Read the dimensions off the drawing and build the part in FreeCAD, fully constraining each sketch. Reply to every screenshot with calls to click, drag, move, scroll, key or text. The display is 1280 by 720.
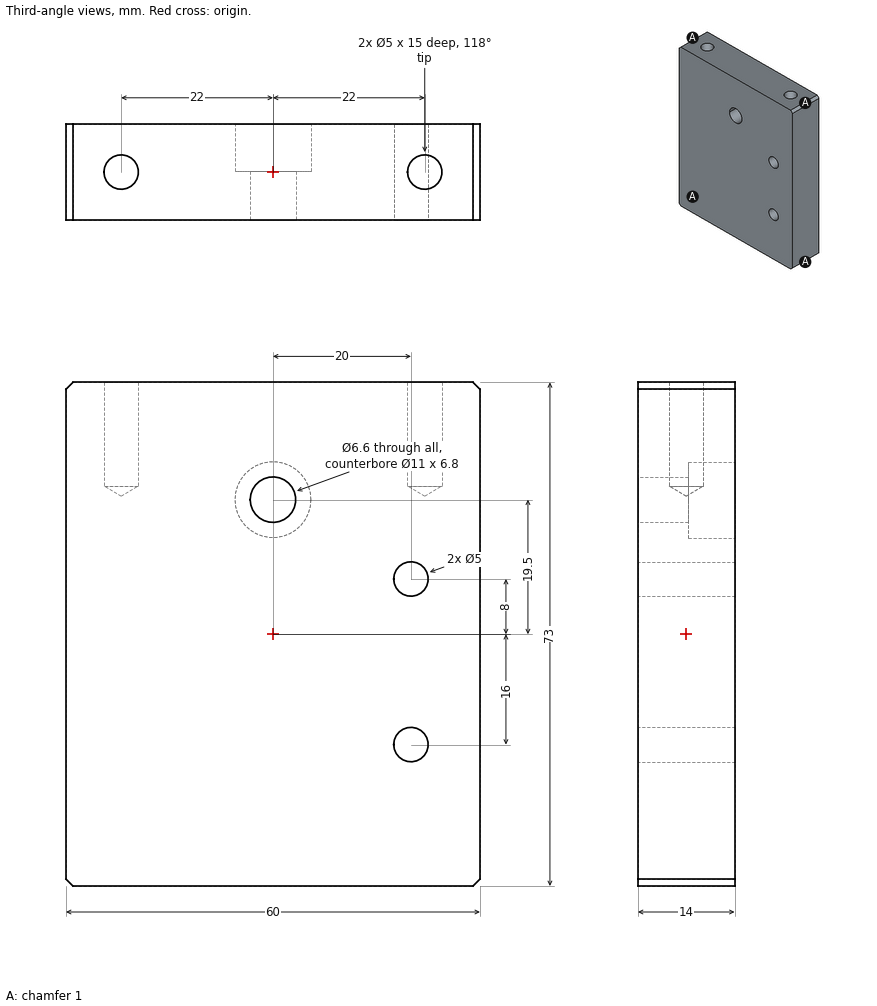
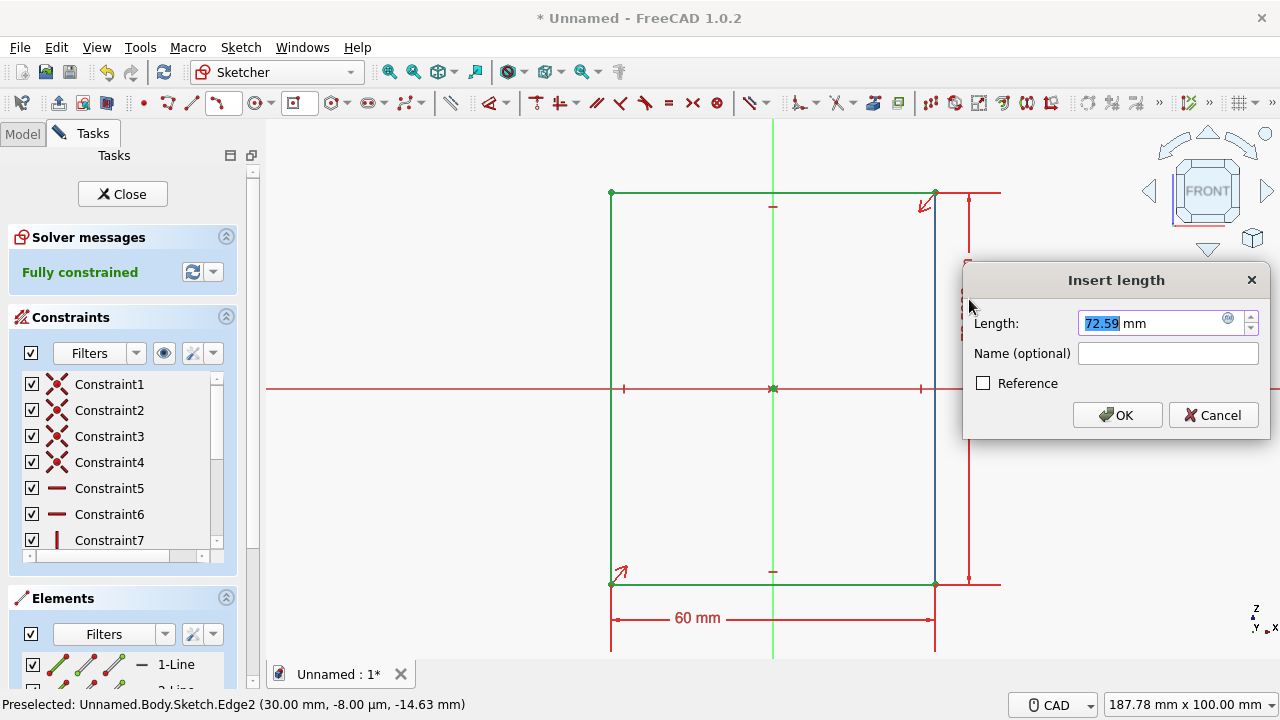
text(73)
key(Return)
key(Escape)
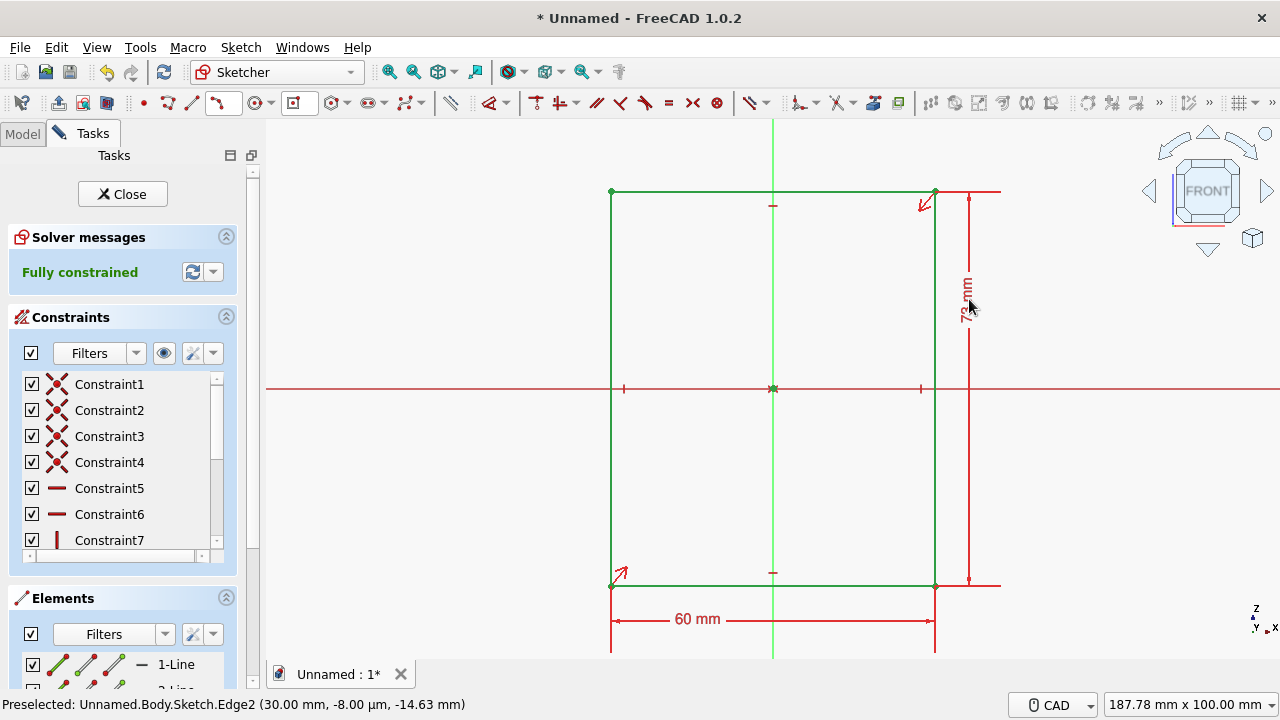
click(123, 194)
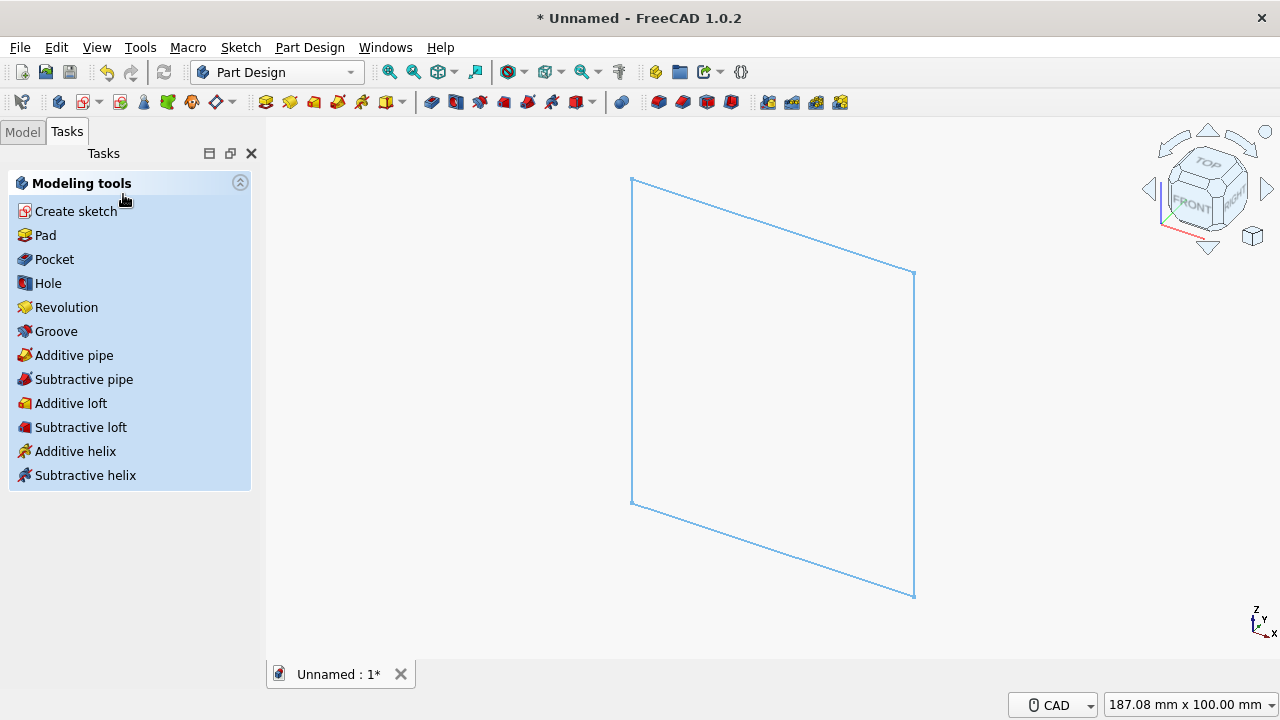
click(266, 102)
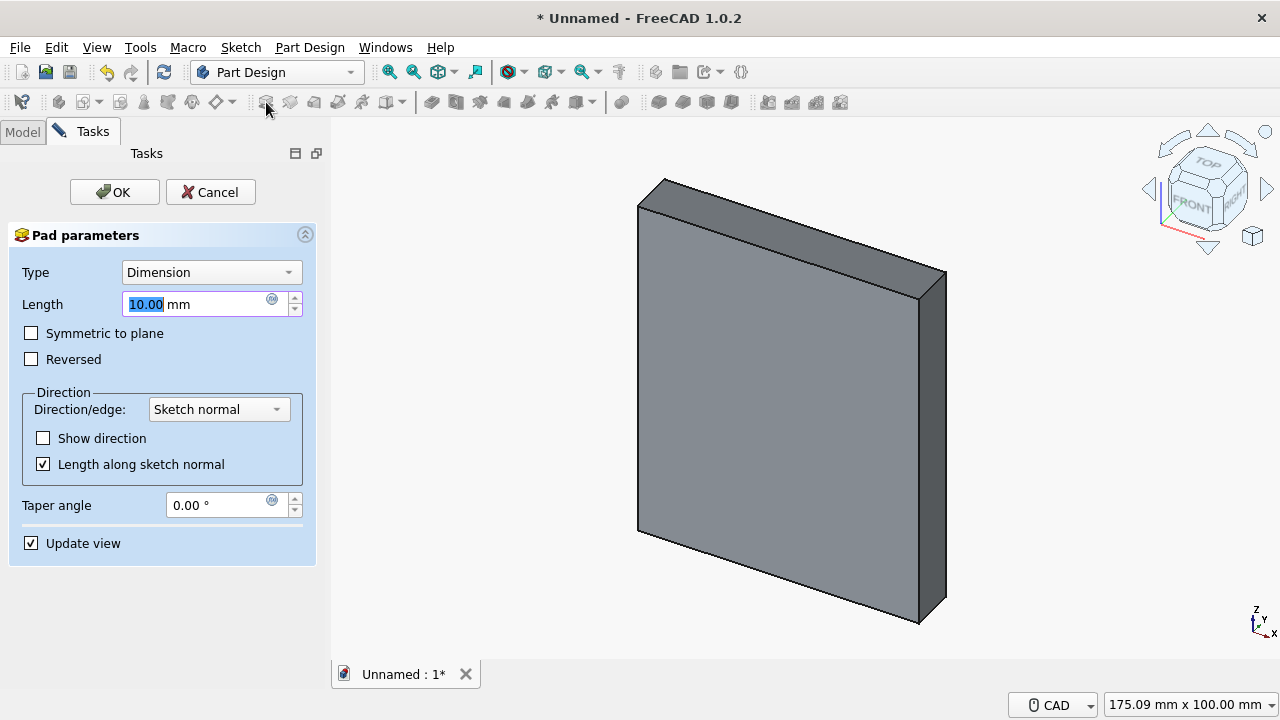
text(14)
key(Tab)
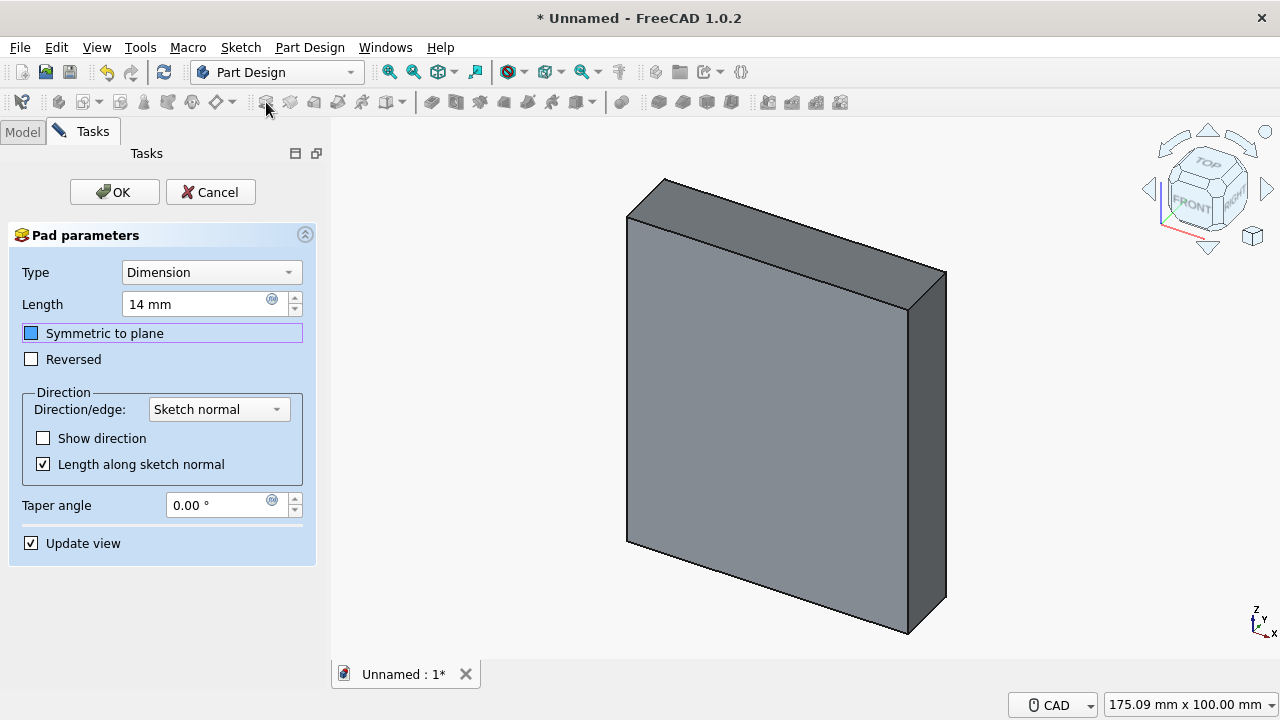
click(30, 333)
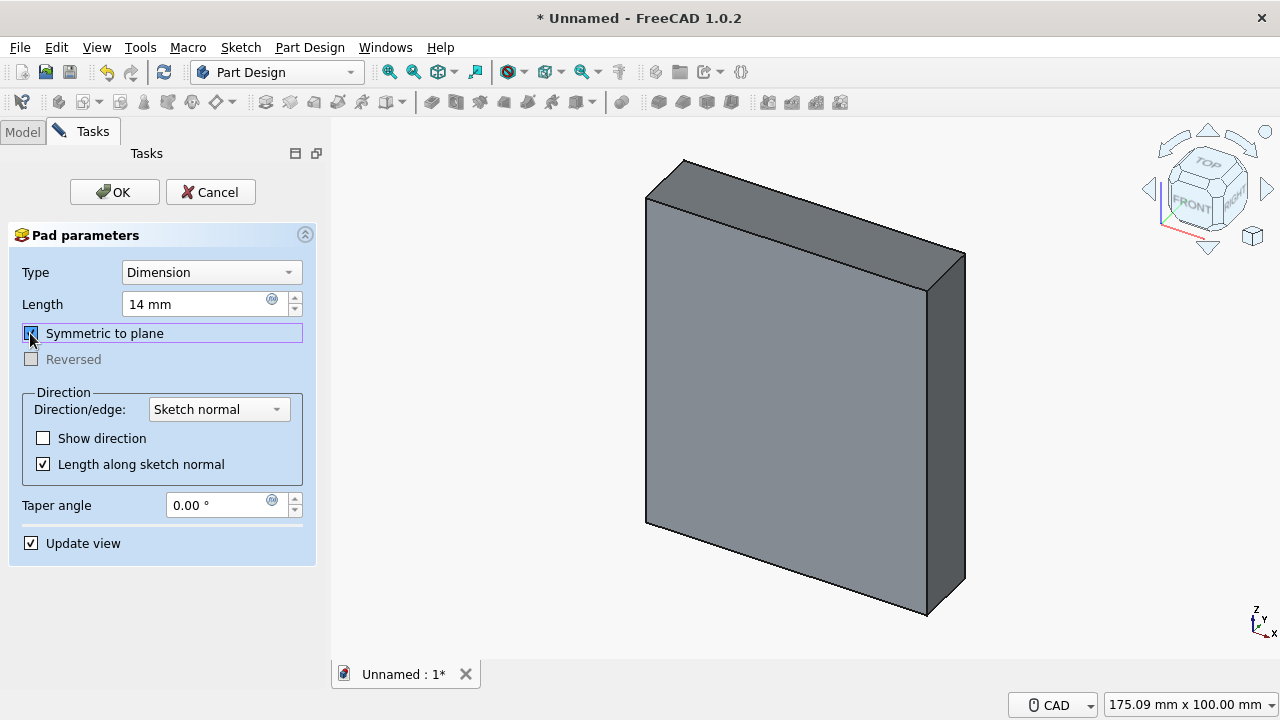
click(115, 192)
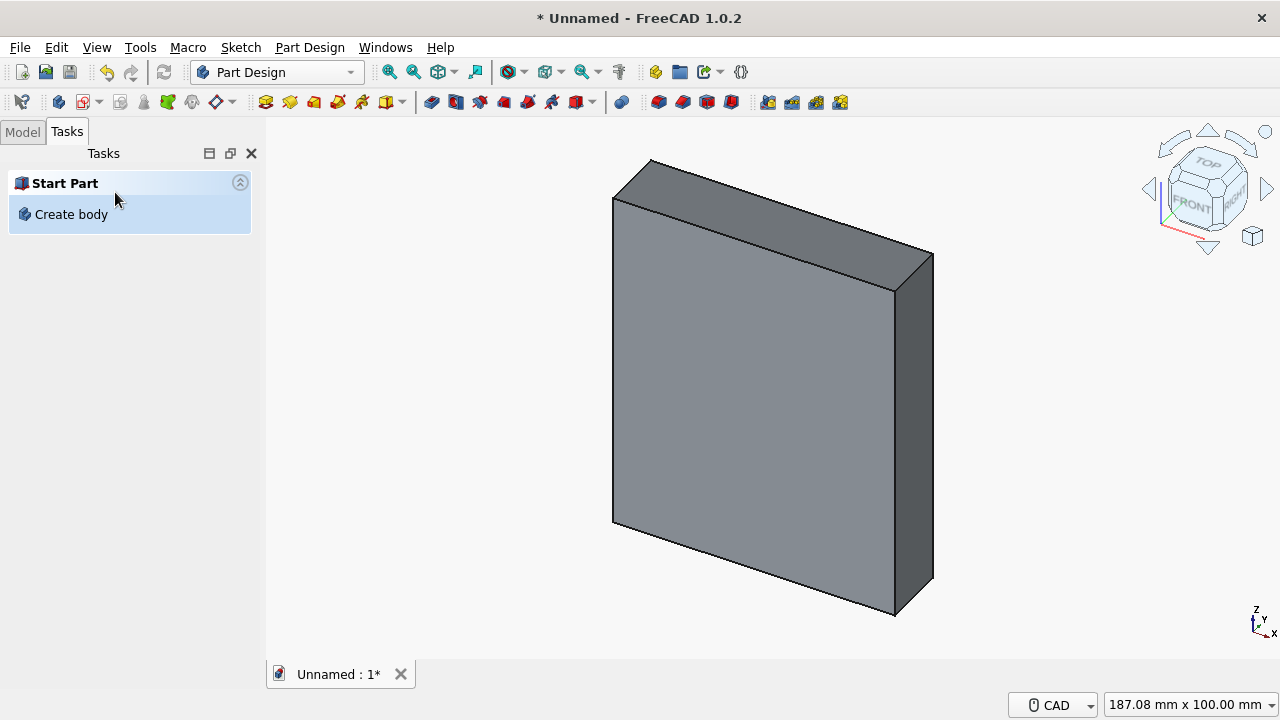
click(853, 252)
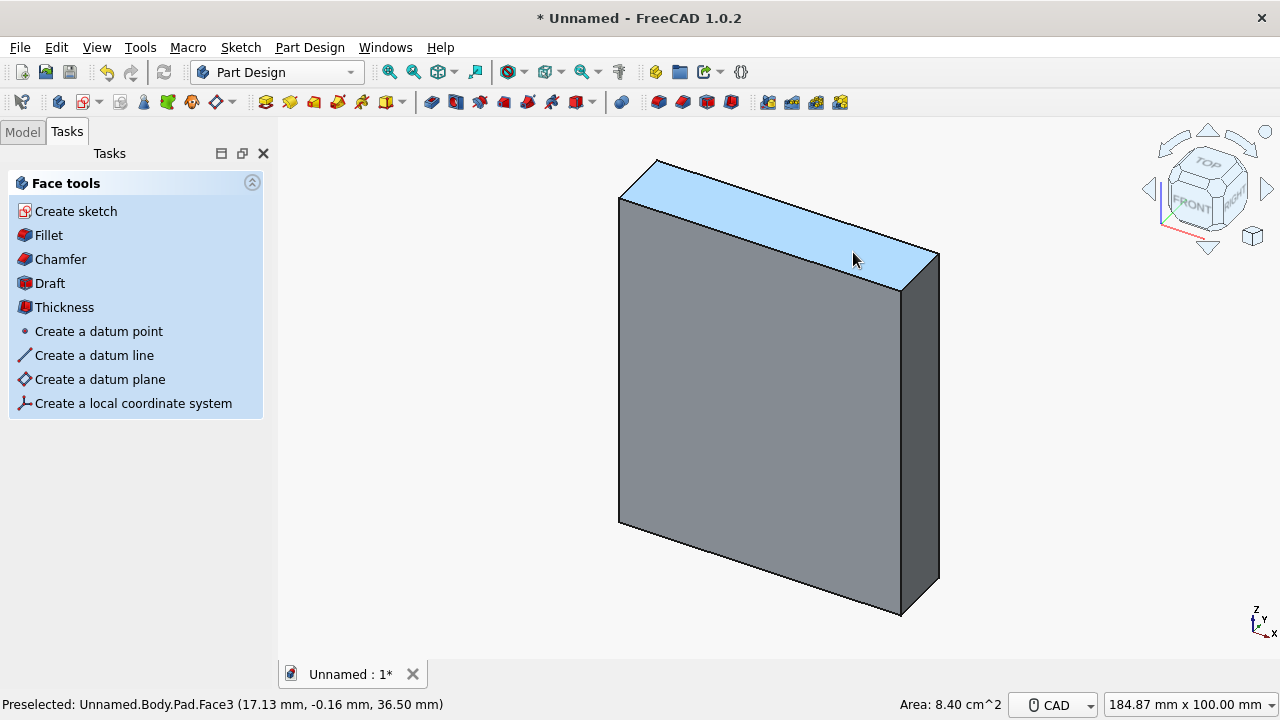
click(84, 102)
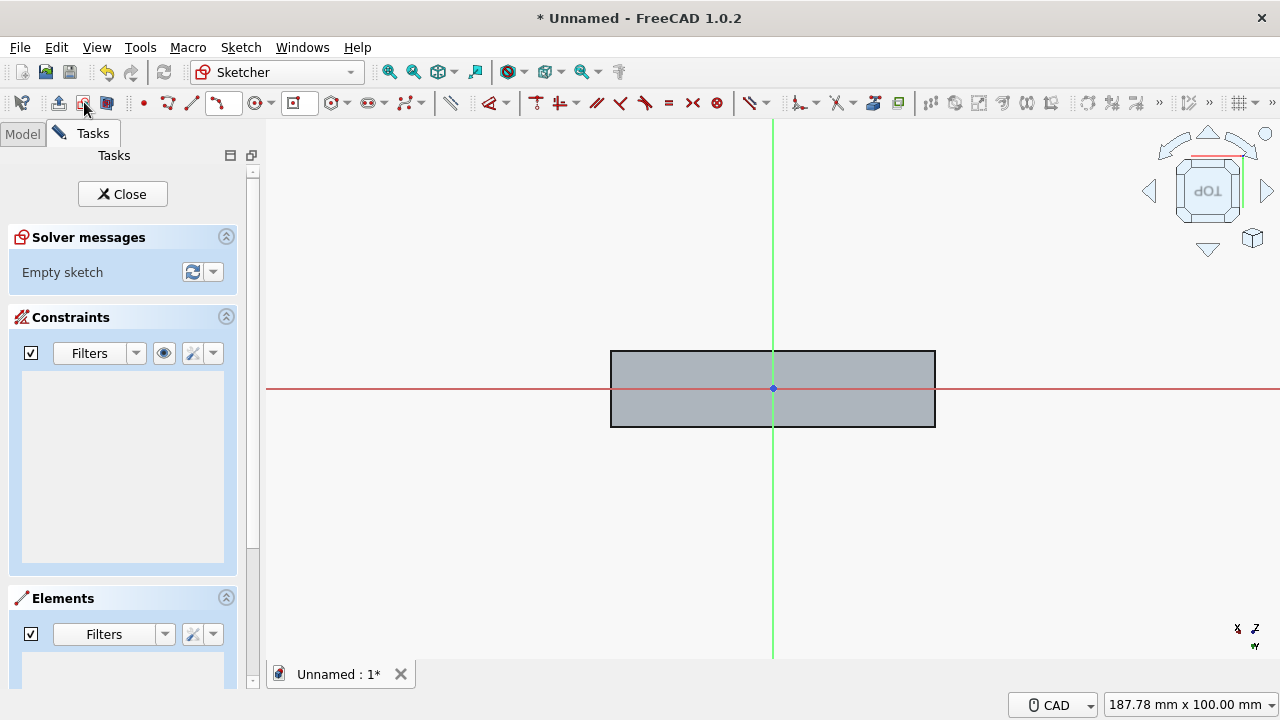
scroll(829, 389, up, 4)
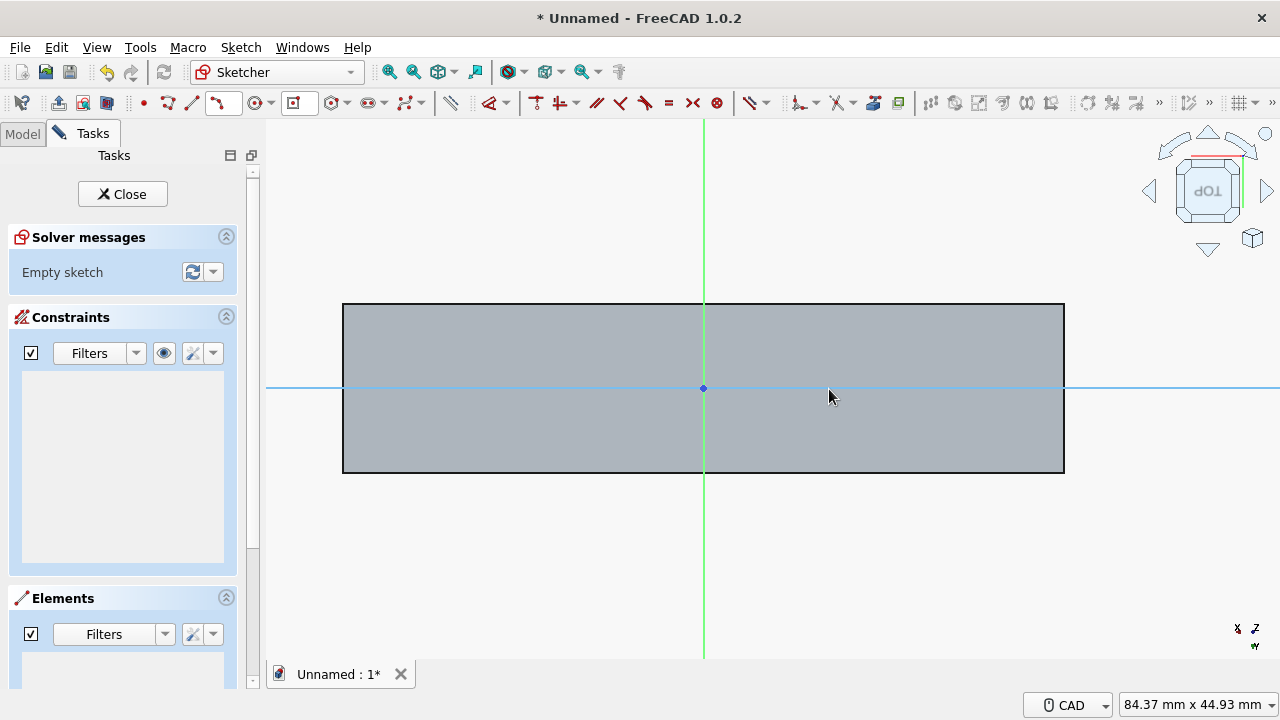
click(256, 104)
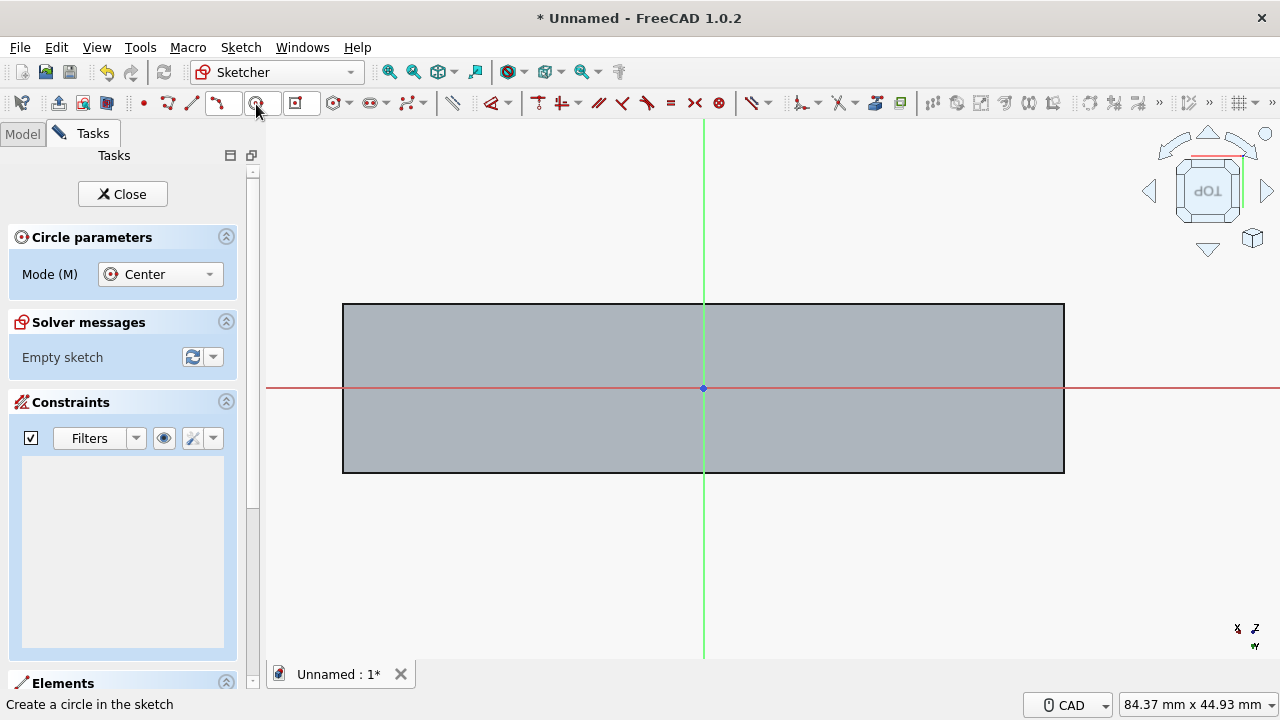
click(439, 388)
click(461, 367)